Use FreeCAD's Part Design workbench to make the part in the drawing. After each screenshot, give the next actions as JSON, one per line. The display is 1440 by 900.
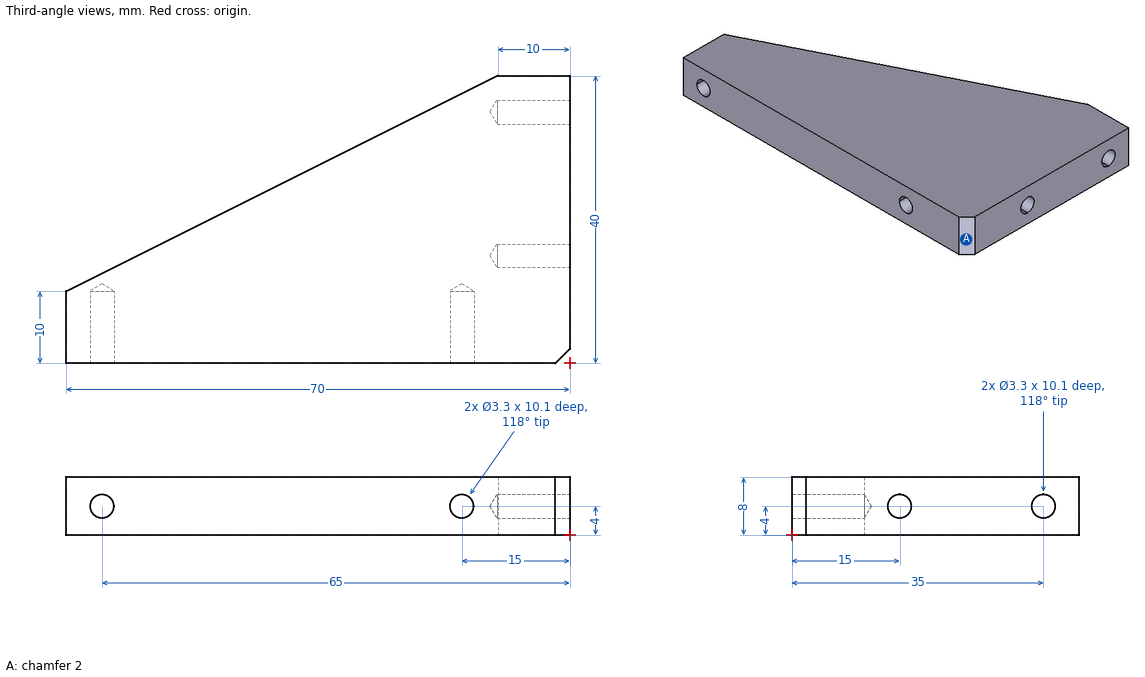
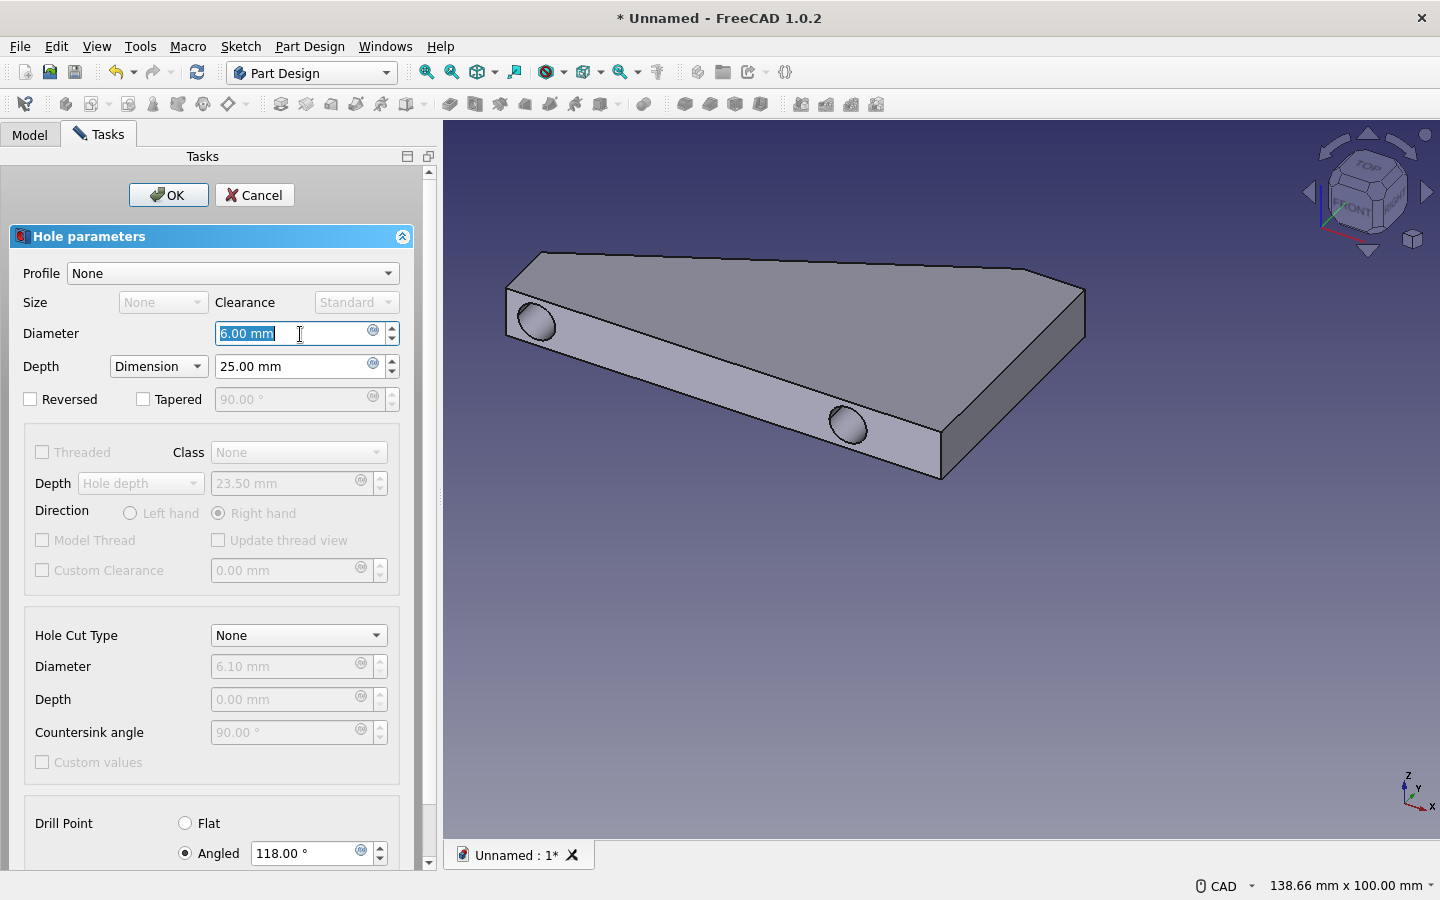
{"action": "type", "text": "3.3"}
{"action": "key", "text": "Tab"}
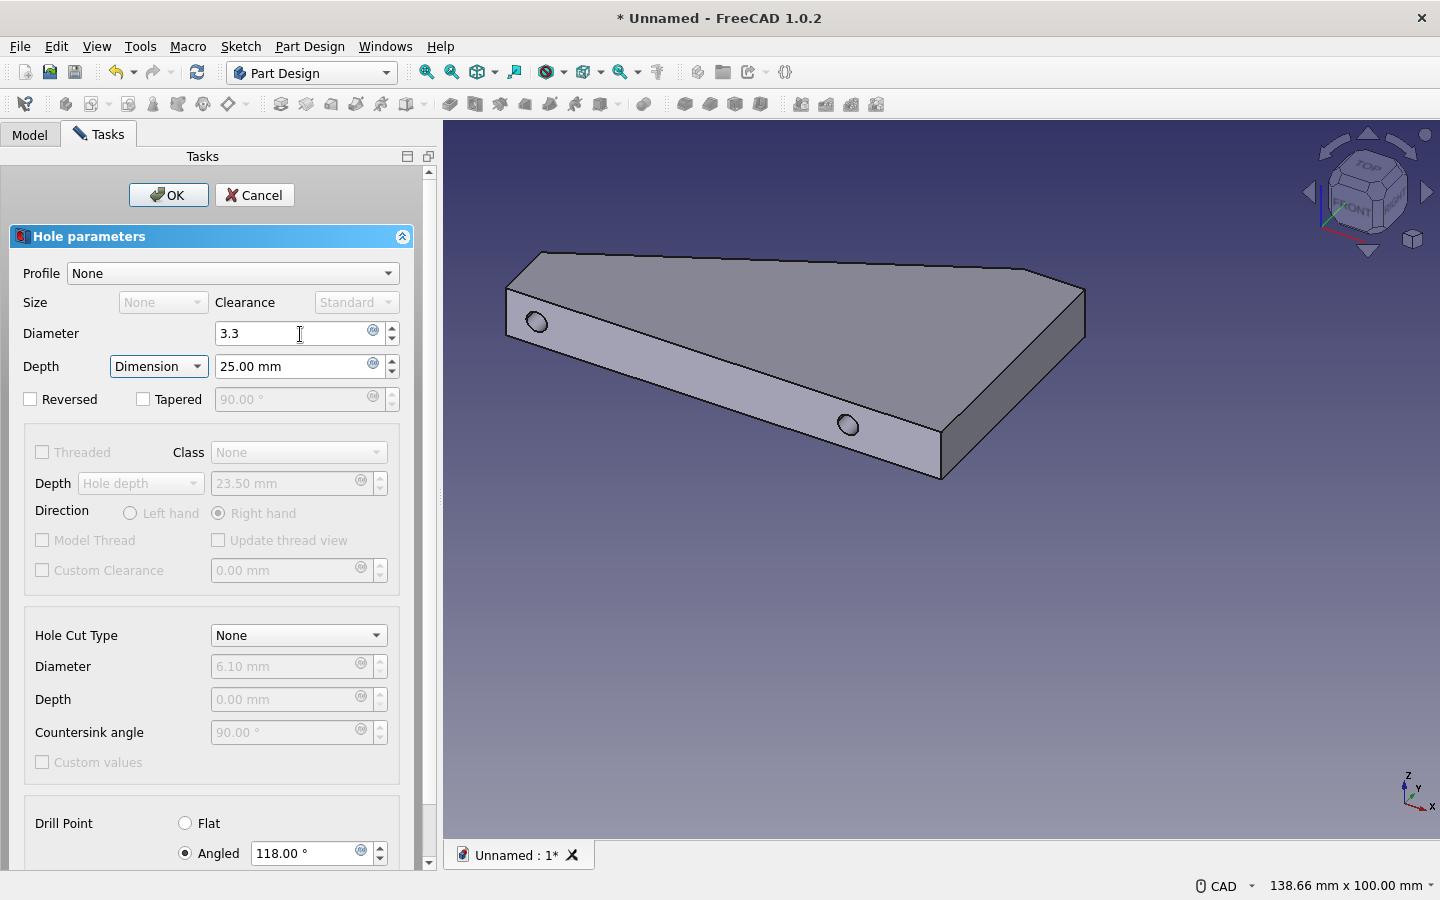
{"action": "triple_click", "coordinate": [300, 366]}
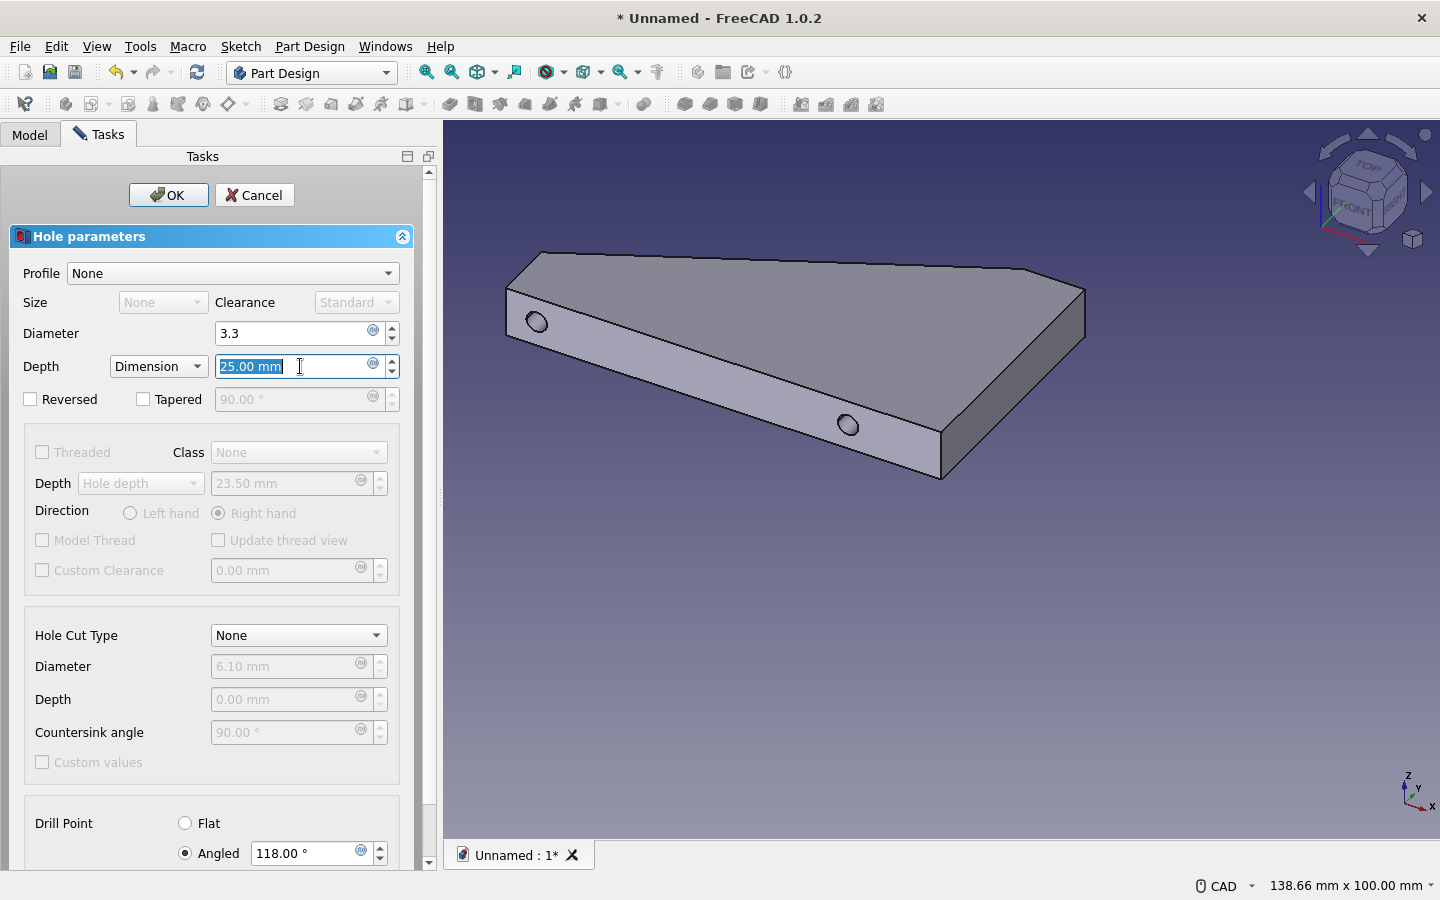
{"action": "type", "text": "10.1"}
{"action": "key", "text": "Tab"}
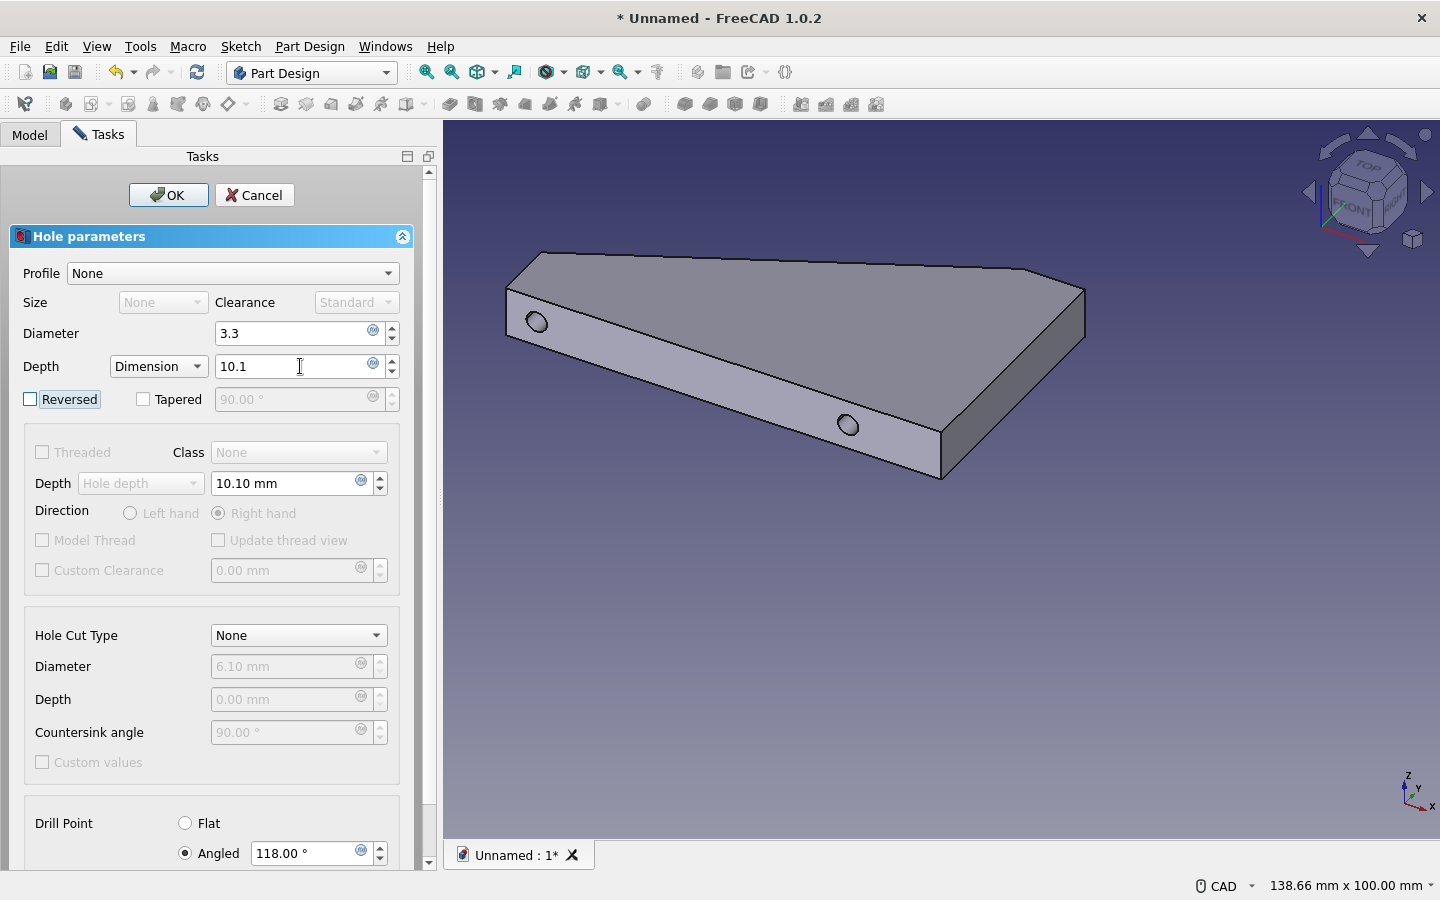
{"action": "left_click", "coordinate": [169, 195]}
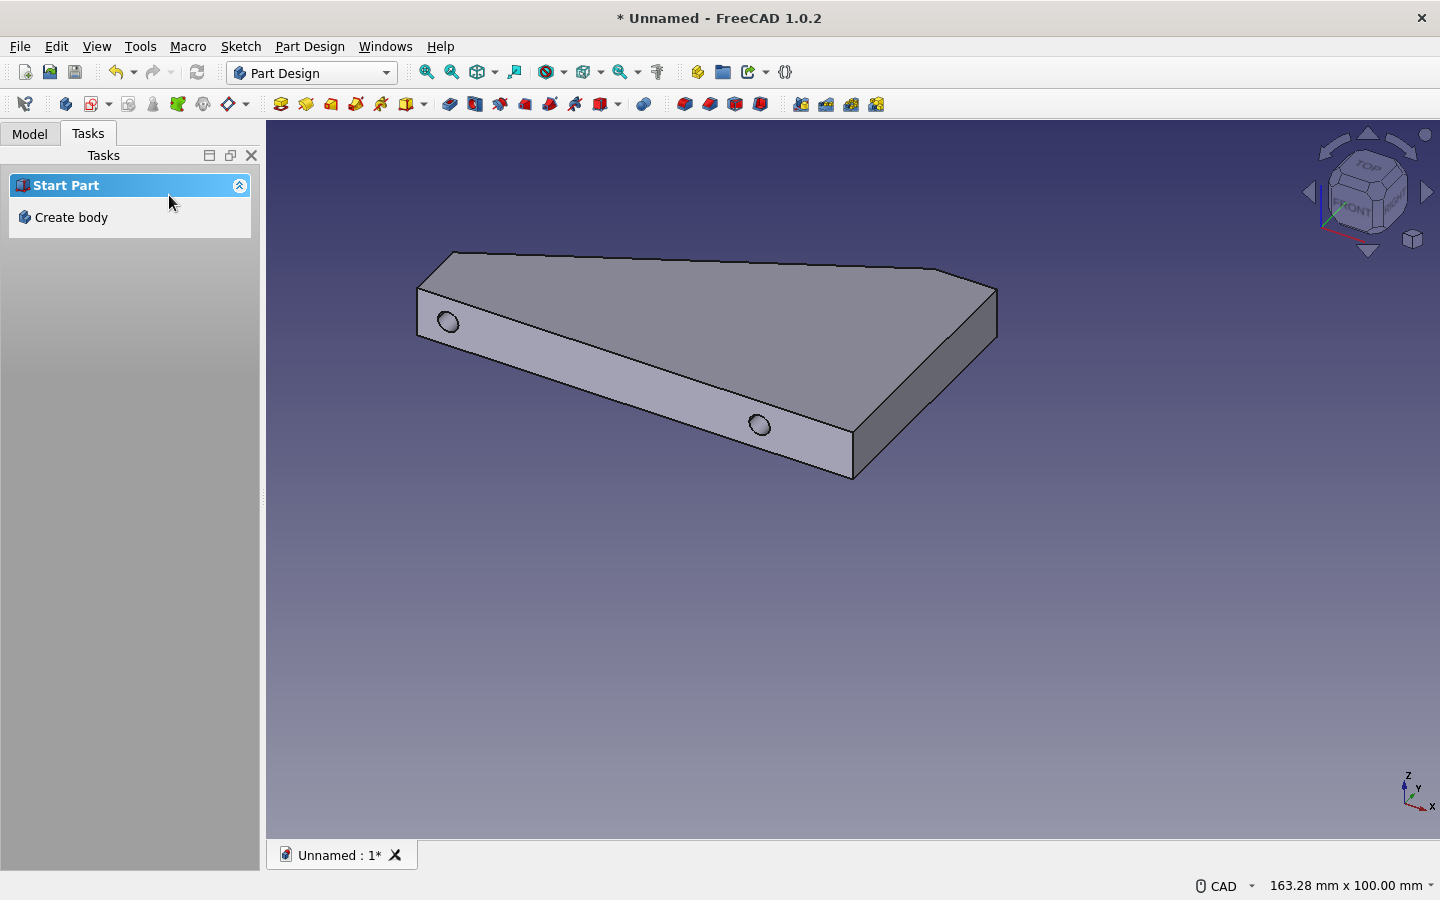
{"action": "left_click", "coordinate": [966, 343]}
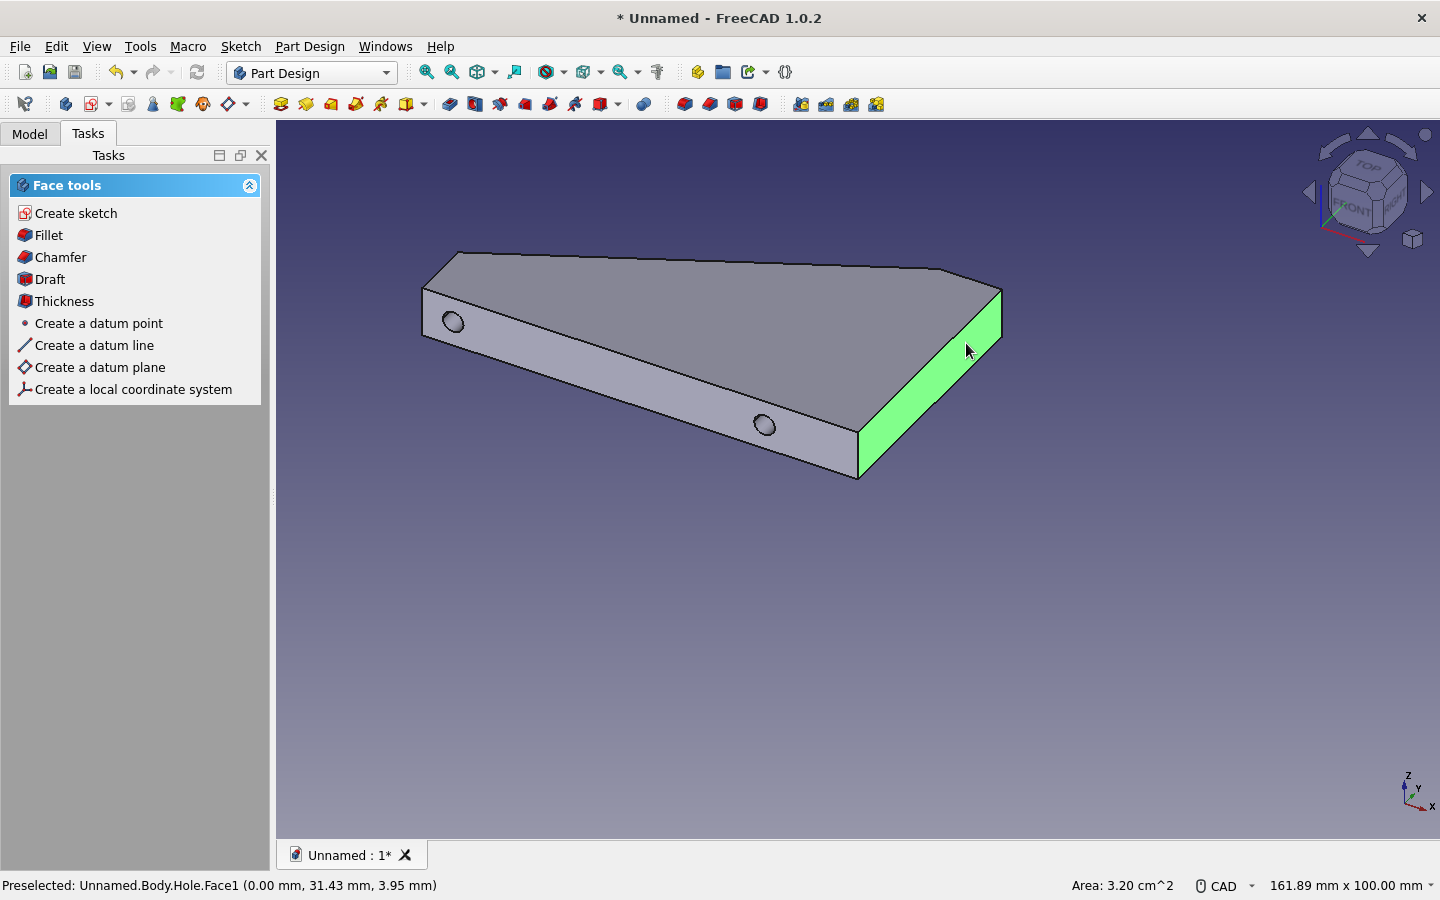
{"action": "left_click", "coordinate": [90, 104]}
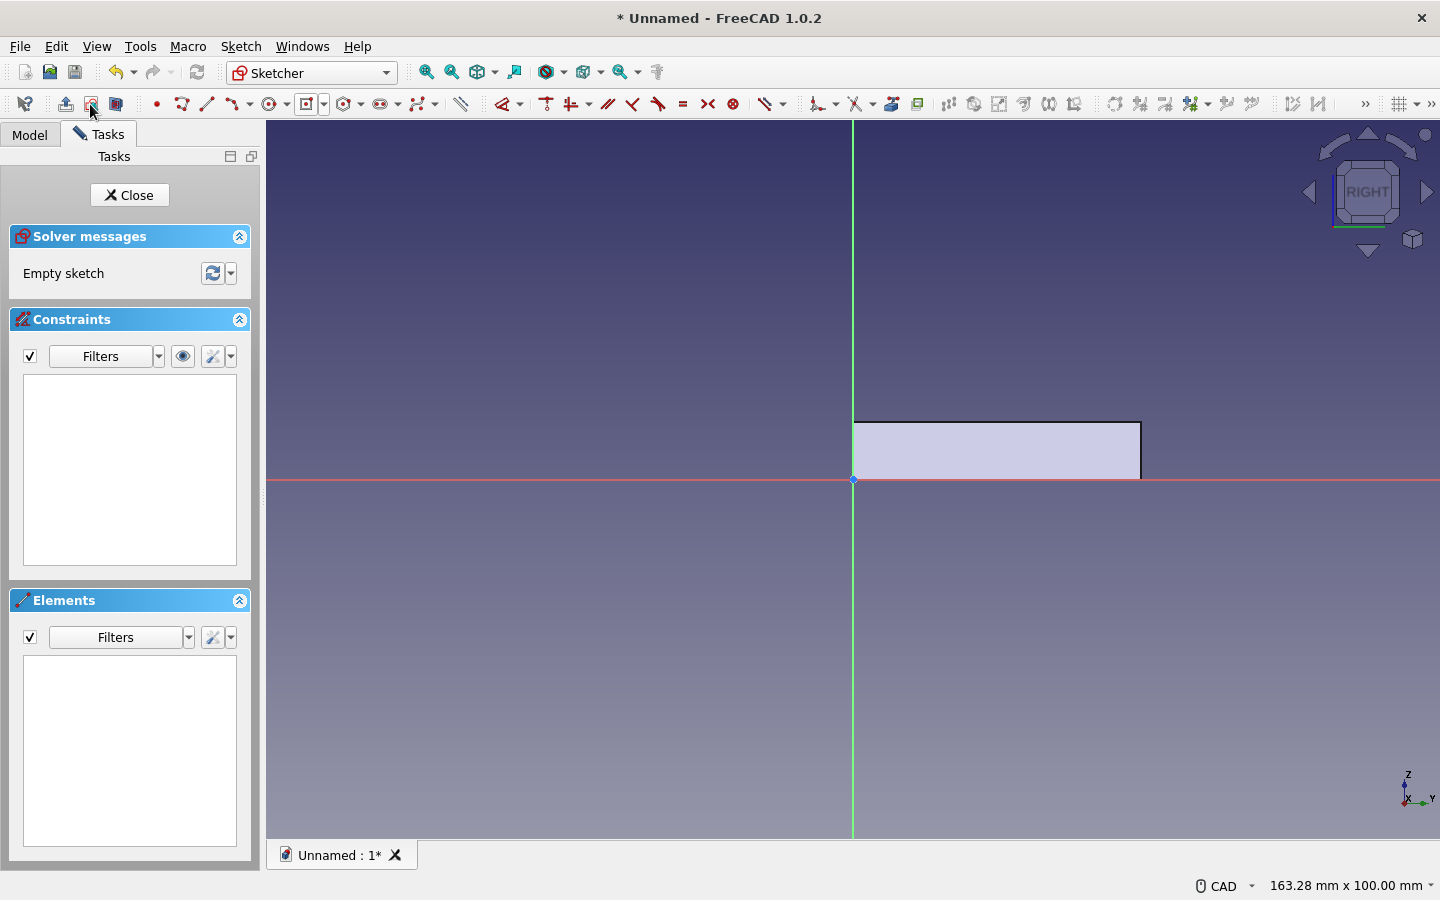
{"action": "scroll", "coordinate": [1101, 447], "scroll_direction": "up", "scroll_amount": 5}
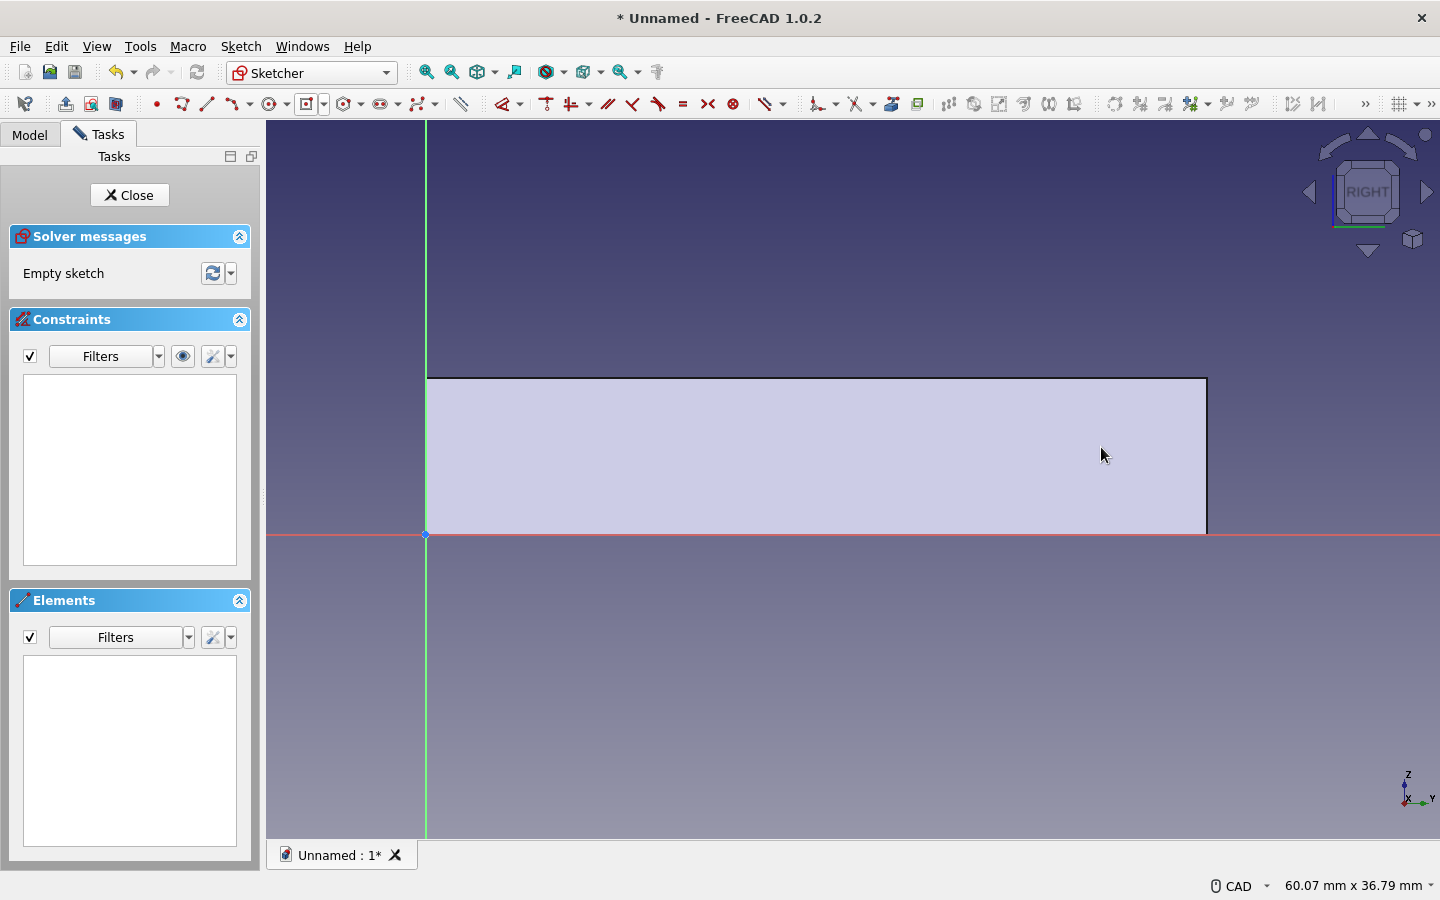
{"action": "left_click", "coordinate": [268, 104]}